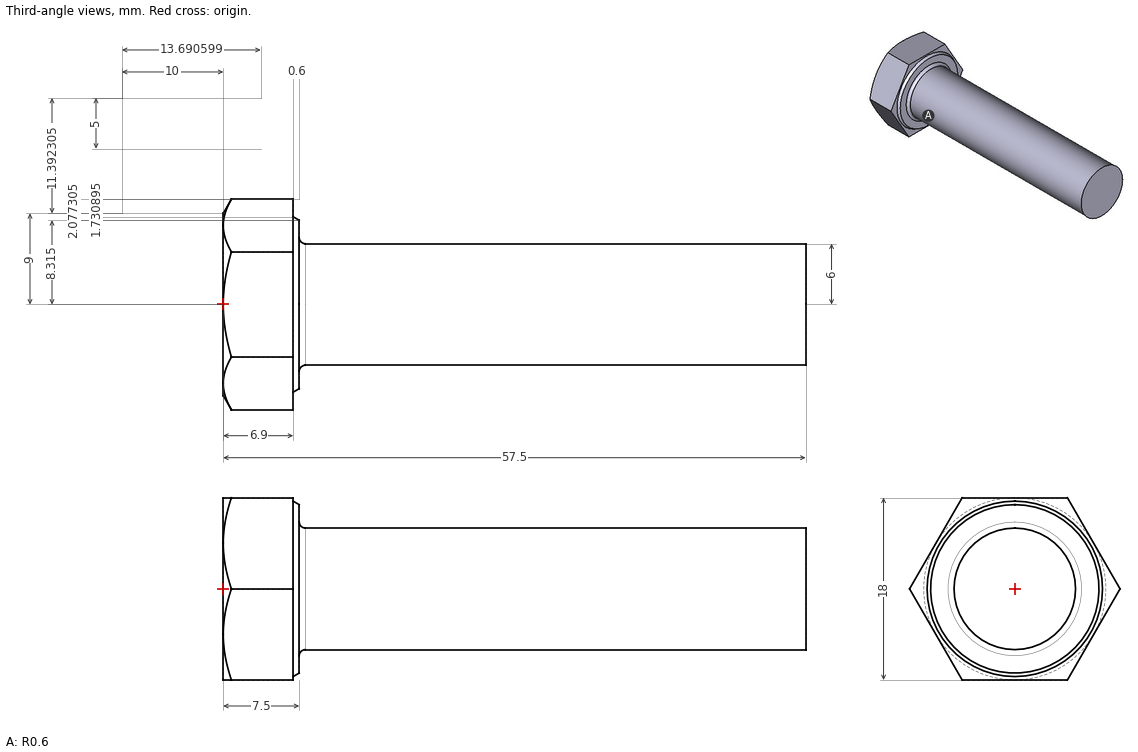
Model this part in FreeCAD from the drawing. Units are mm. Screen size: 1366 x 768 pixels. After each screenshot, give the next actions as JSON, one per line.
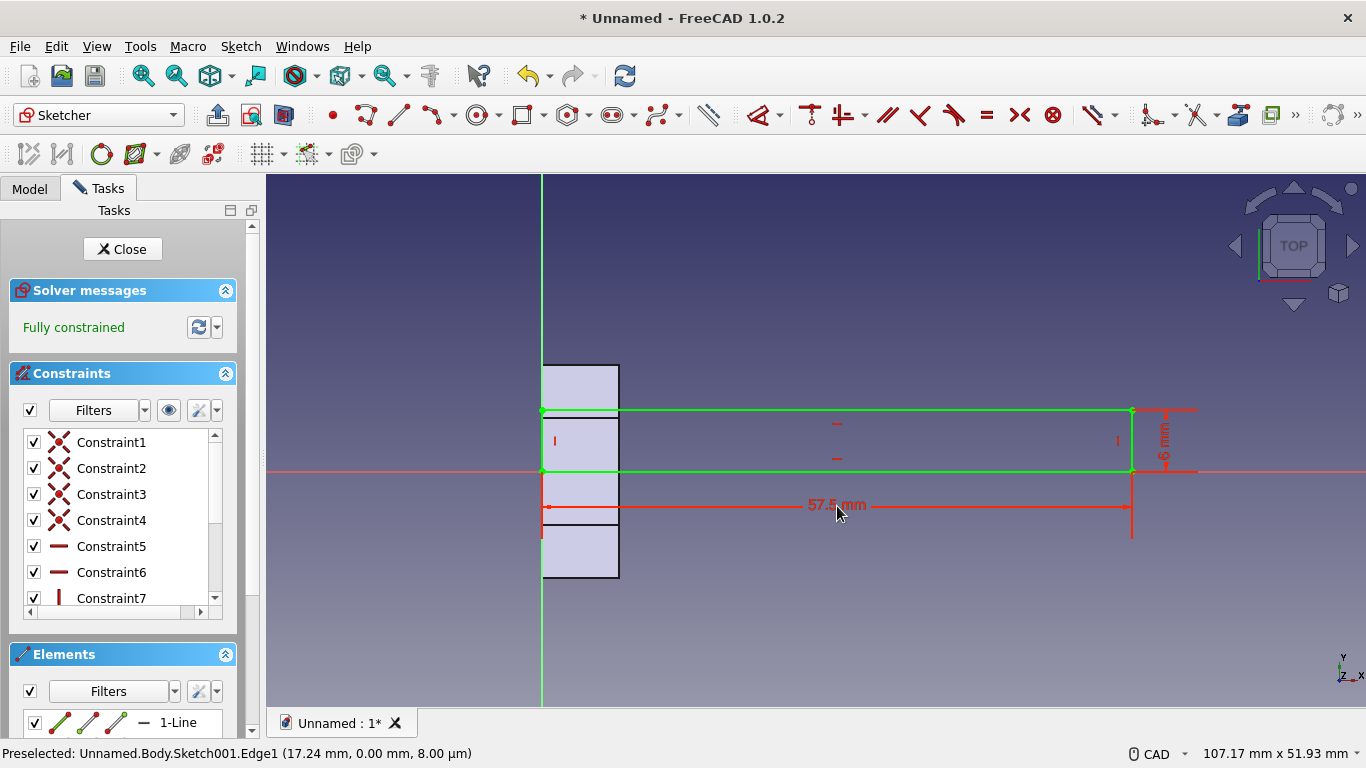
{"action": "left_click", "coordinate": [123, 249]}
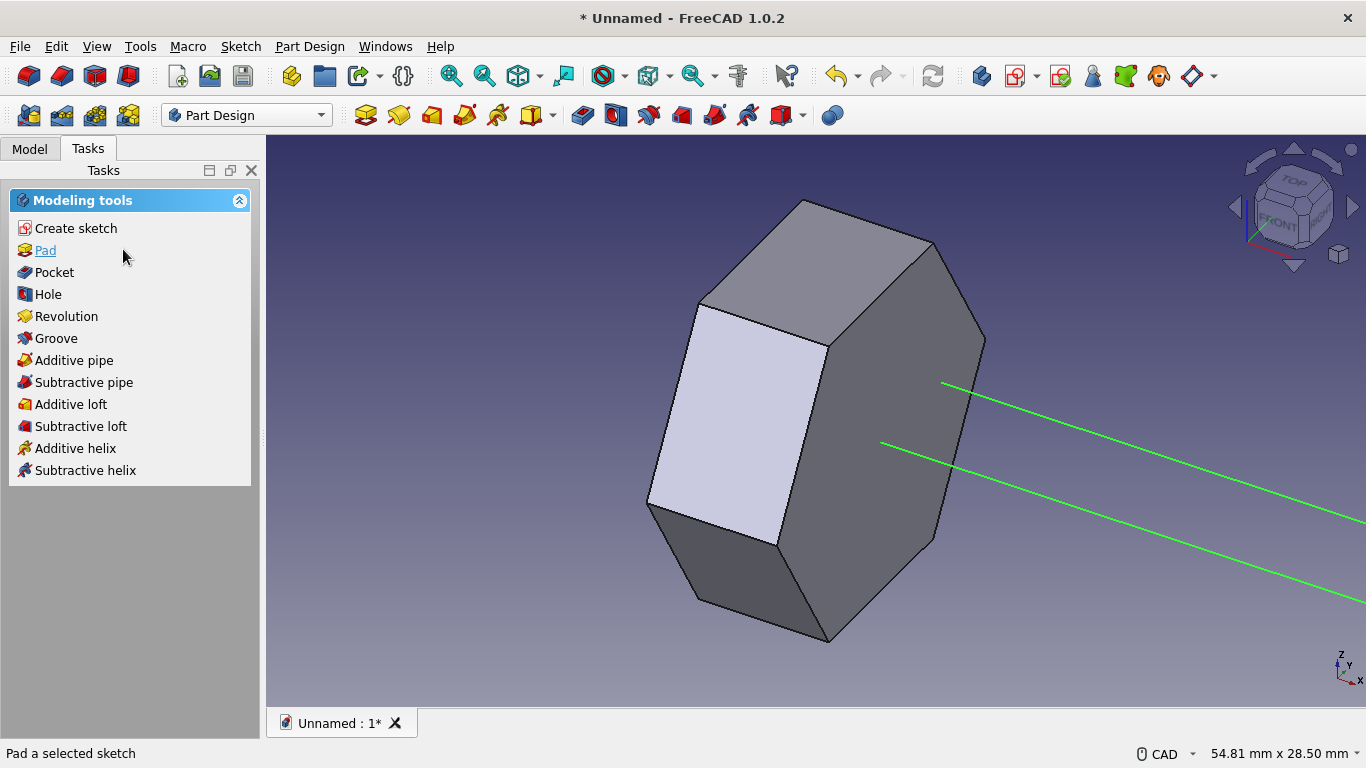
{"action": "left_click", "coordinate": [399, 116]}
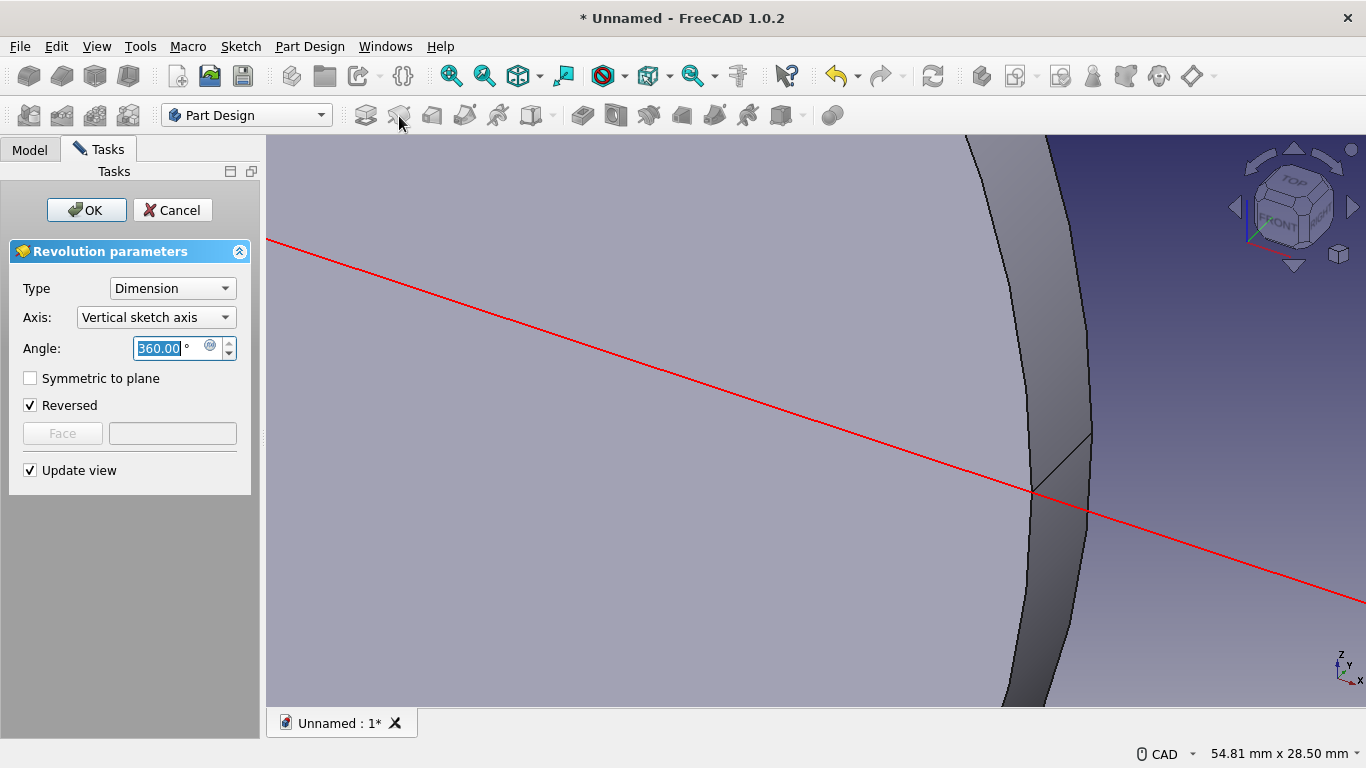
{"action": "left_click", "coordinate": [157, 318]}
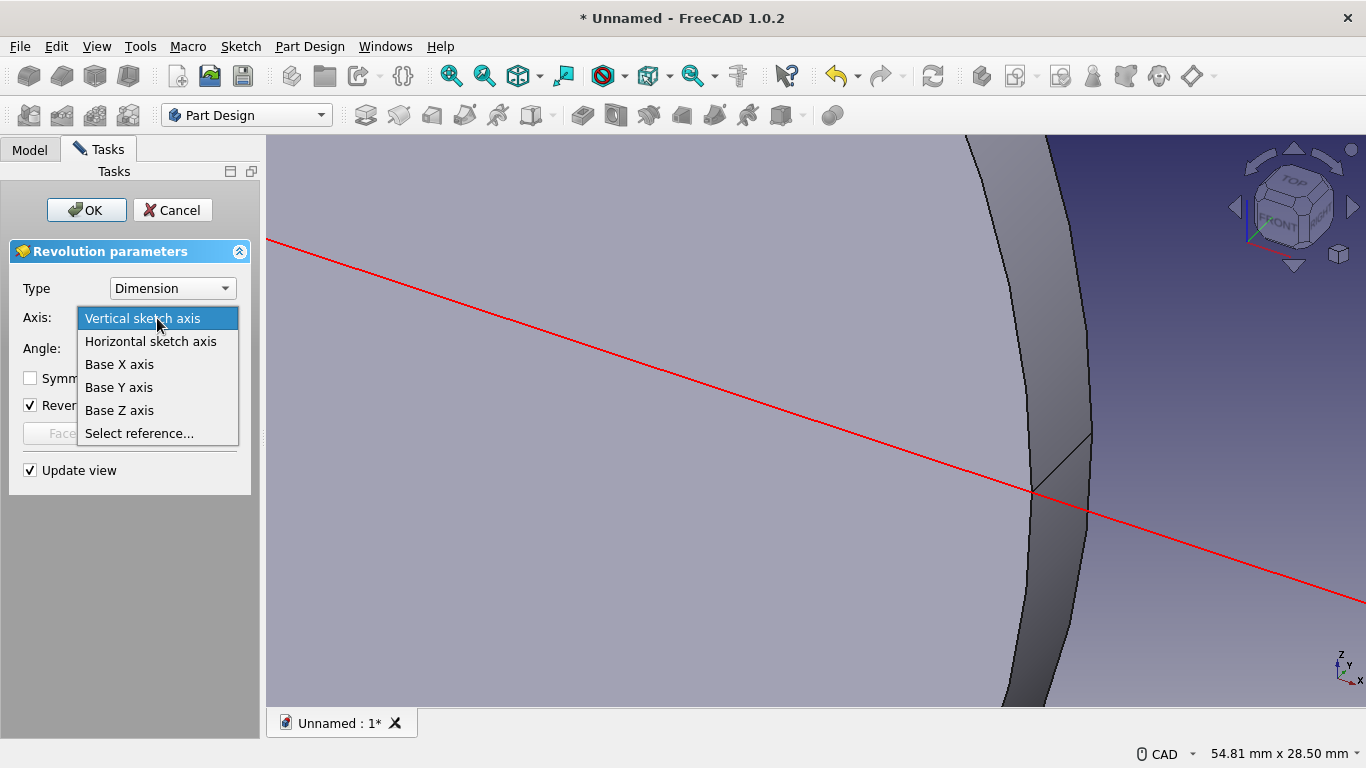
{"action": "left_click", "coordinate": [156, 342]}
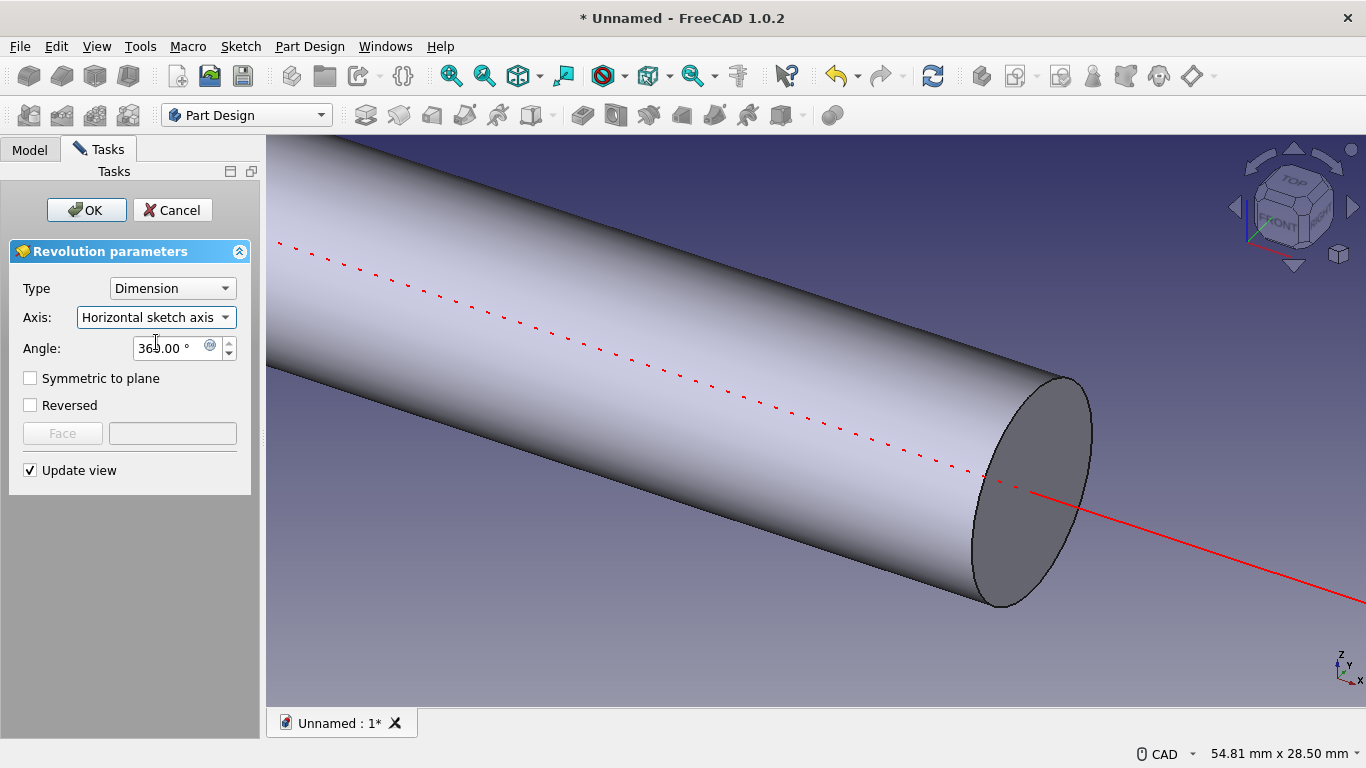
{"action": "left_click", "coordinate": [87, 210]}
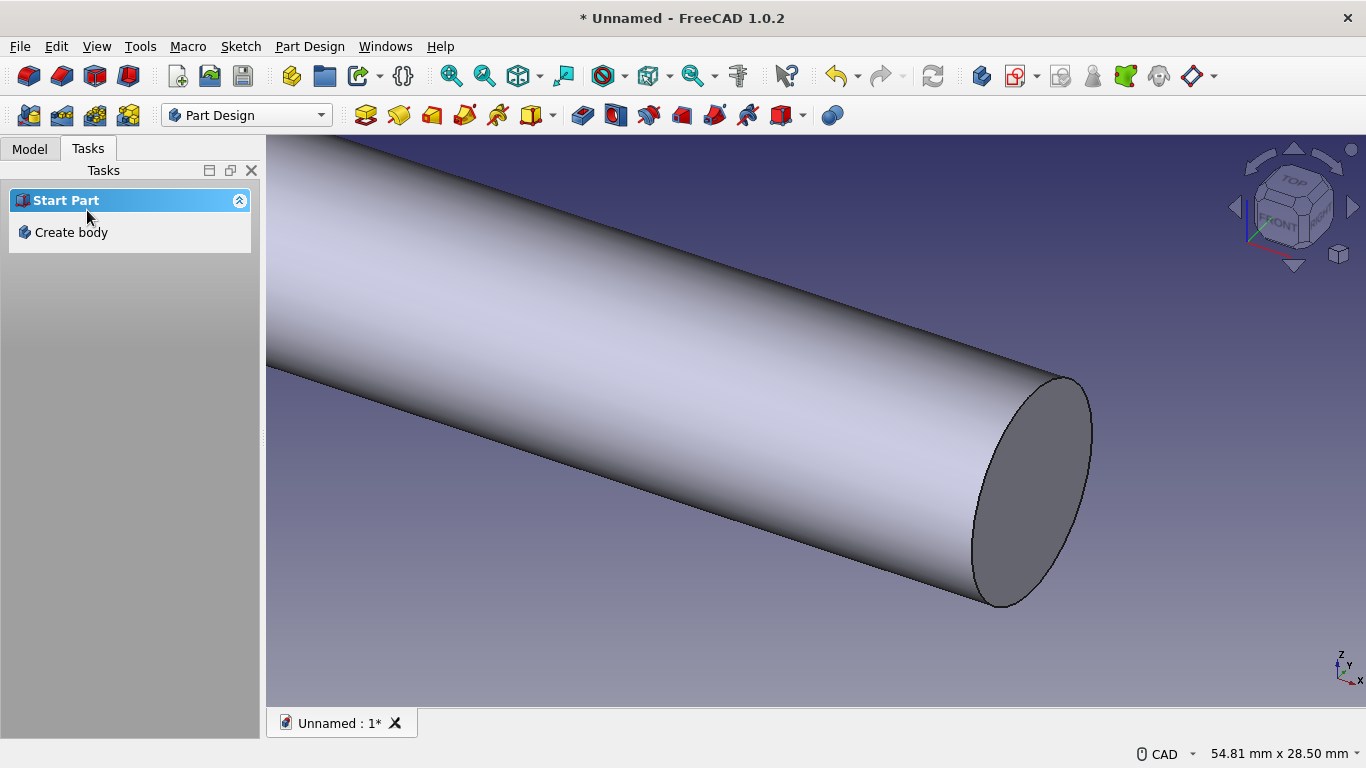
{"action": "left_click", "coordinate": [452, 76]}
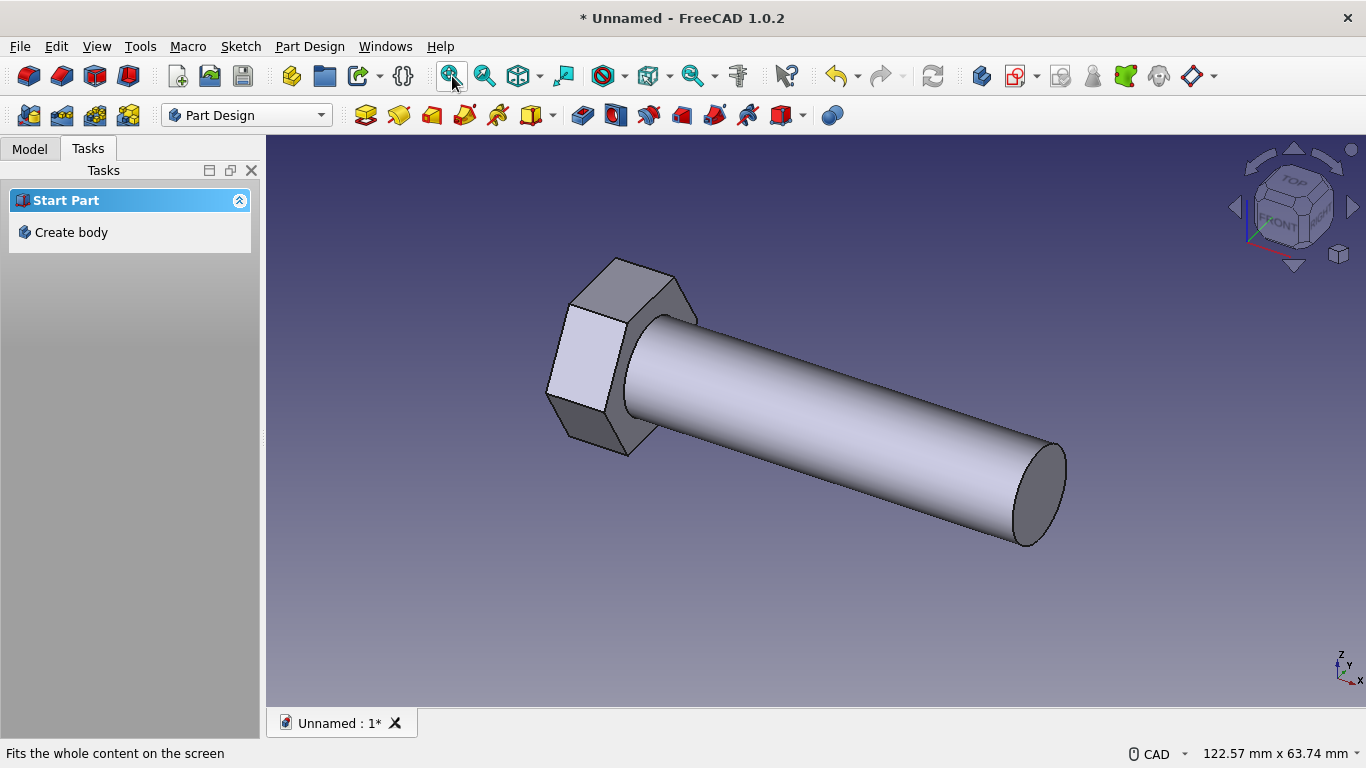
{"action": "left_click", "coordinate": [1014, 76]}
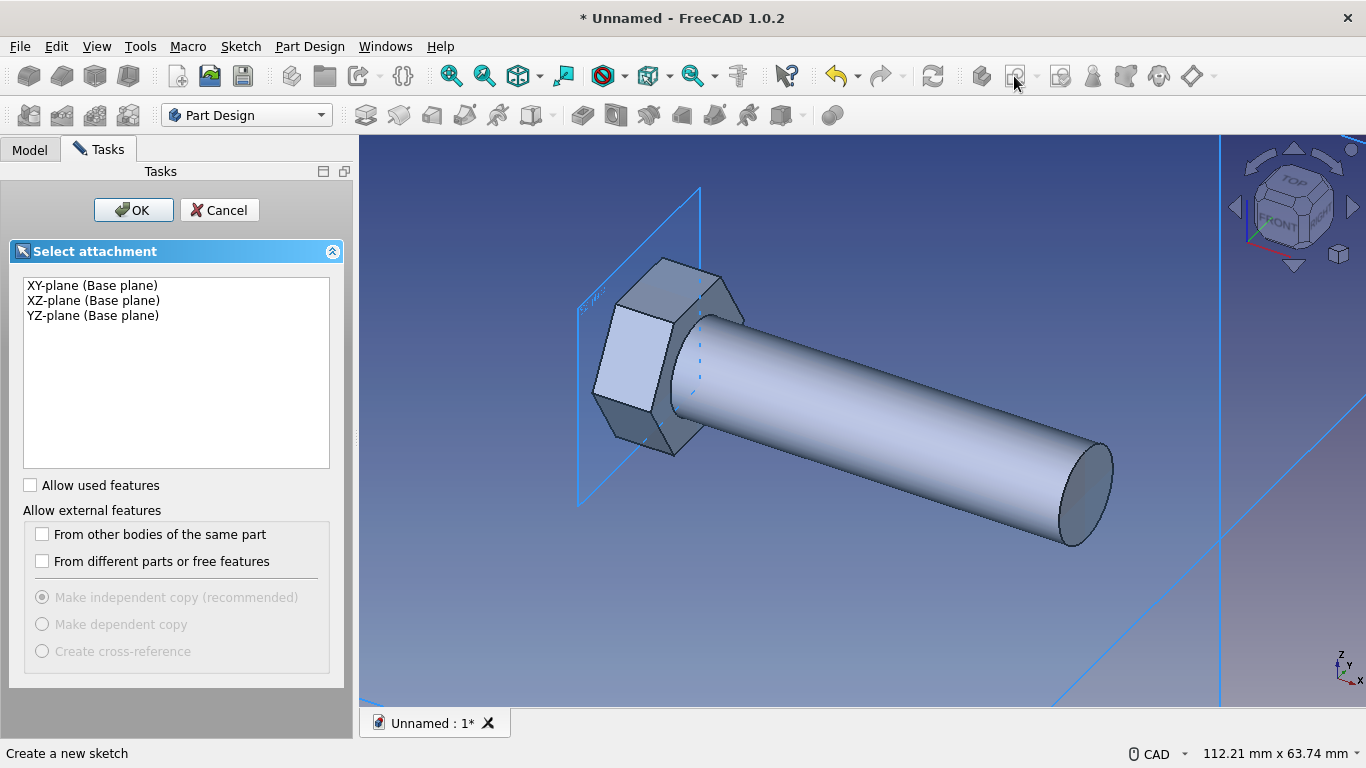
{"action": "left_click", "coordinate": [84, 286]}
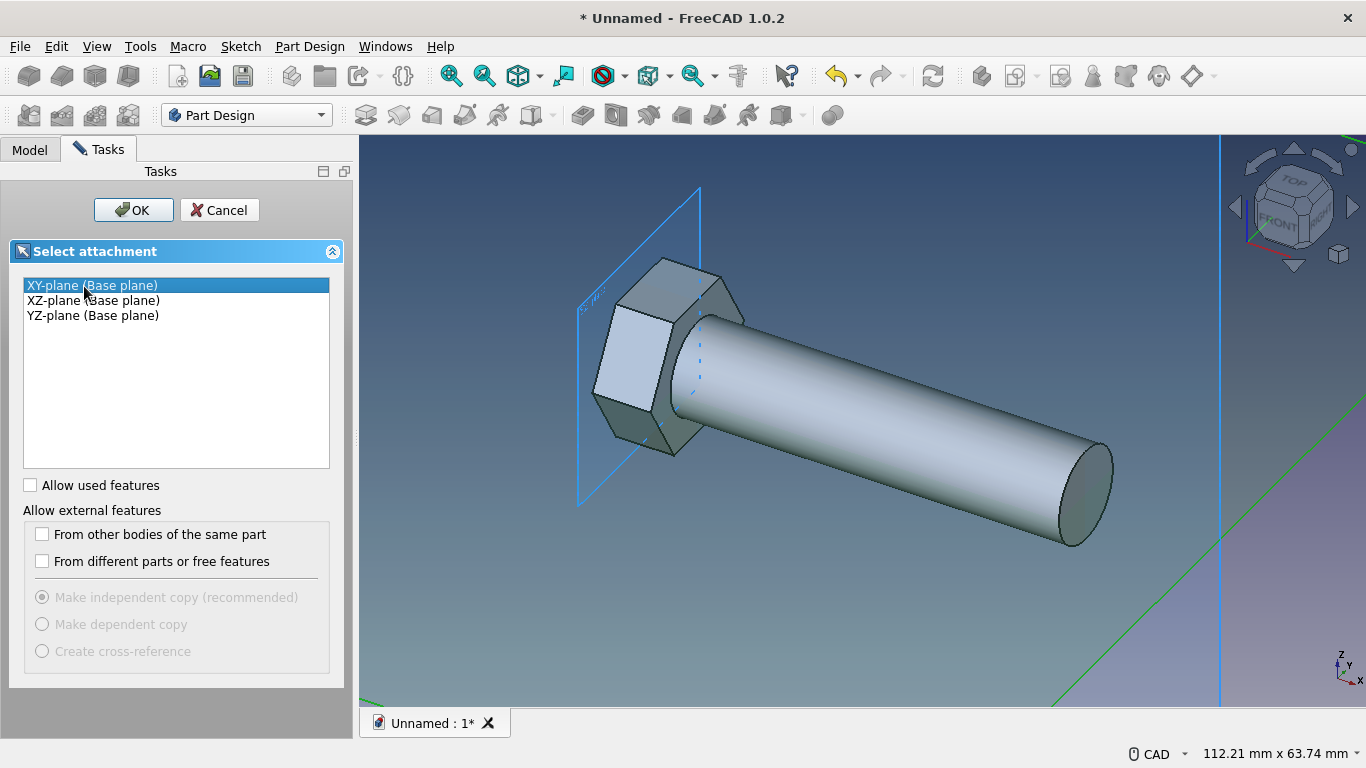
{"action": "left_click", "coordinate": [134, 210]}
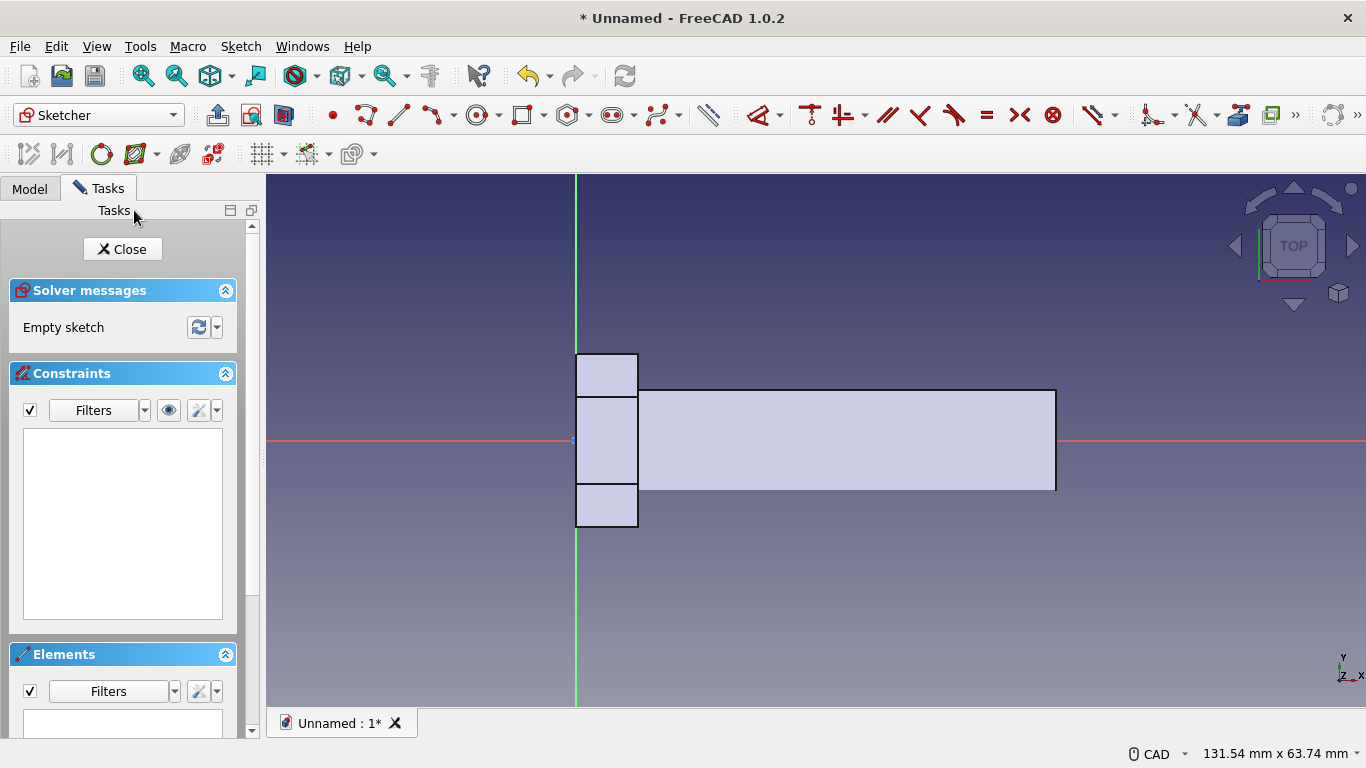
{"action": "left_click", "coordinate": [284, 116]}